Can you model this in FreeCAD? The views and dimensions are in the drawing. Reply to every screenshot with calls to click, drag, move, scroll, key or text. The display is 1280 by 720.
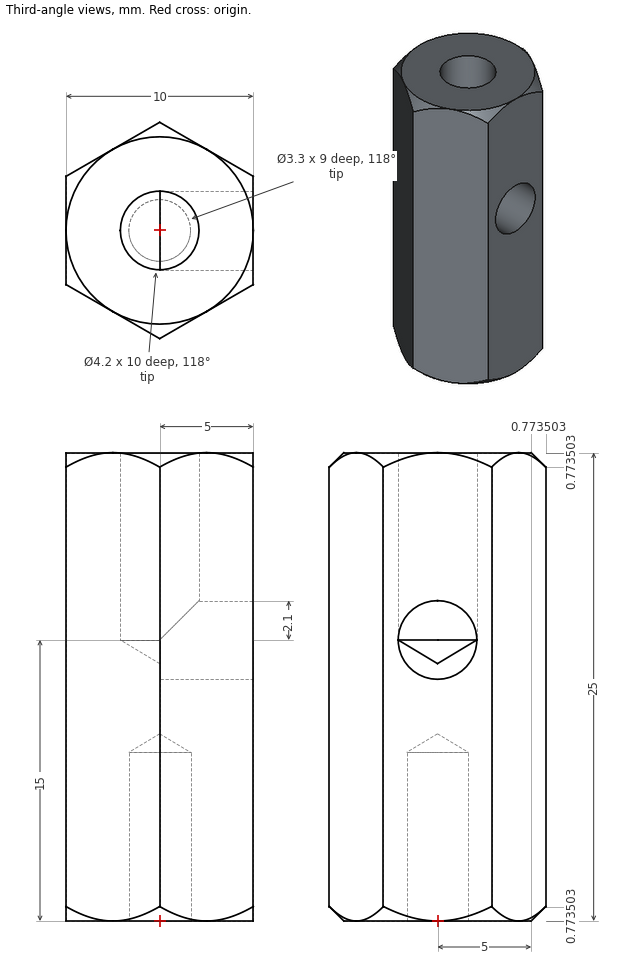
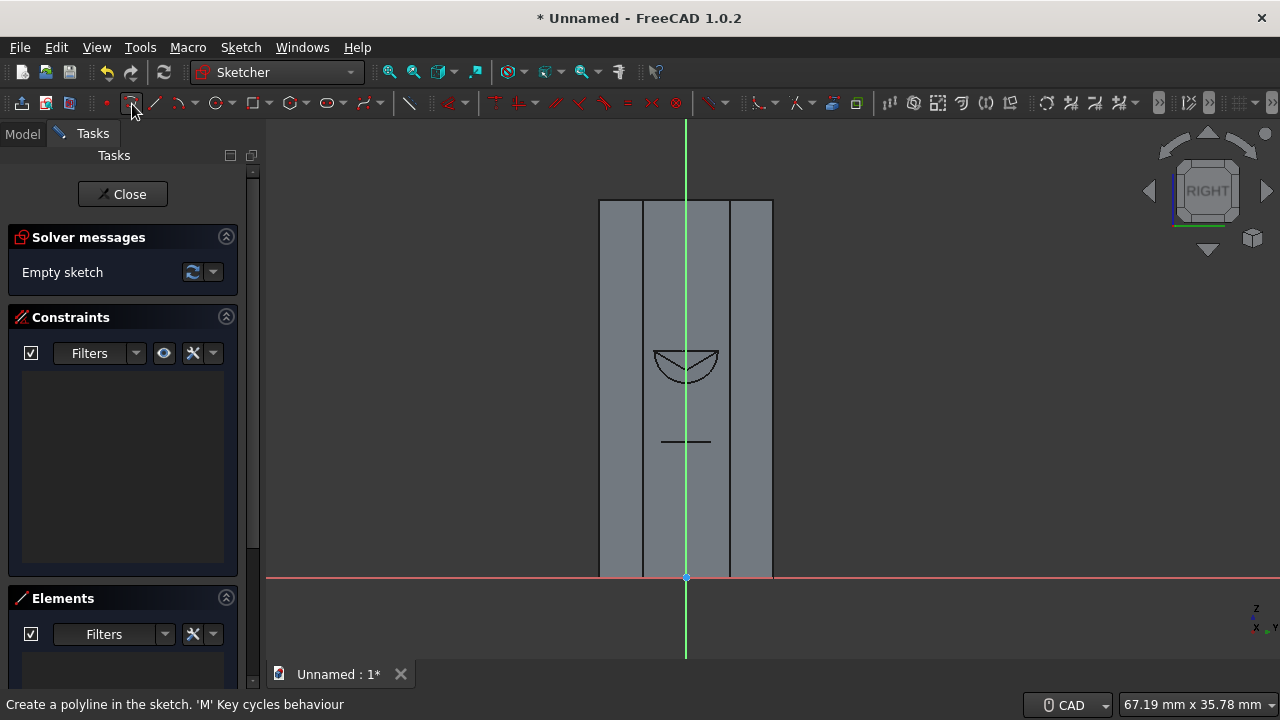
click(773, 212)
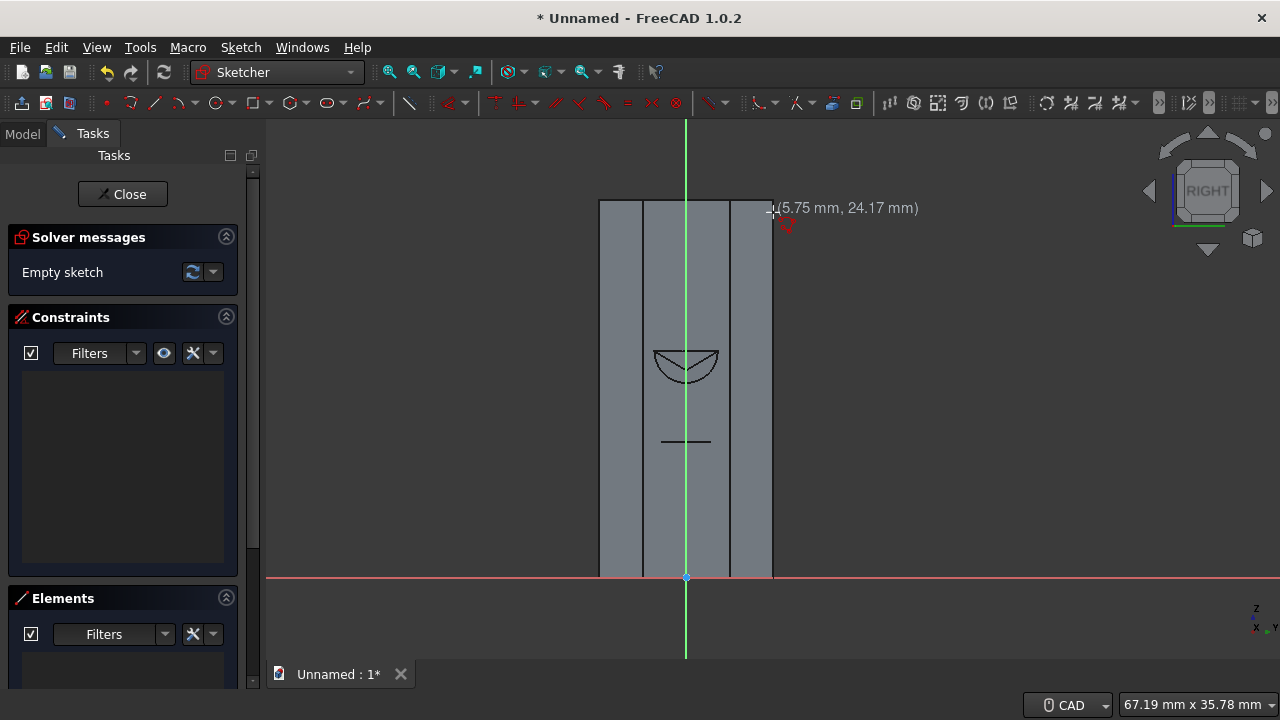
scroll(773, 200, up, 2)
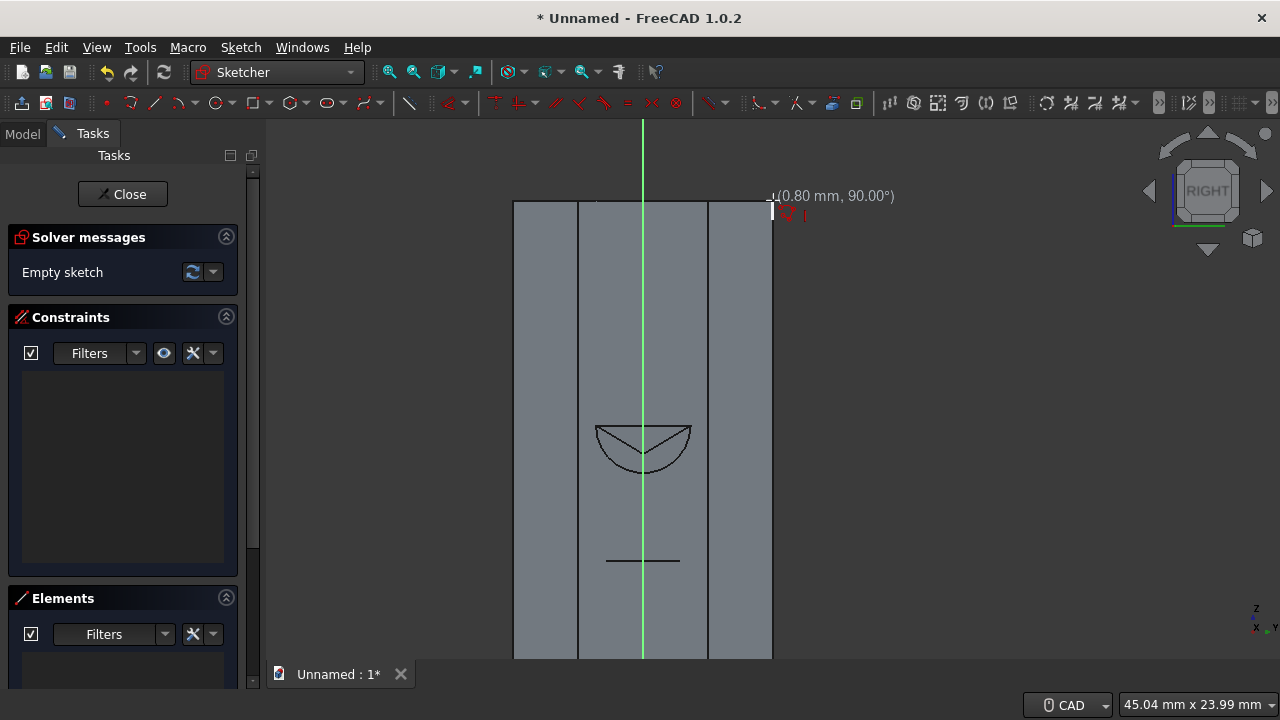
click(773, 201)
click(756, 201)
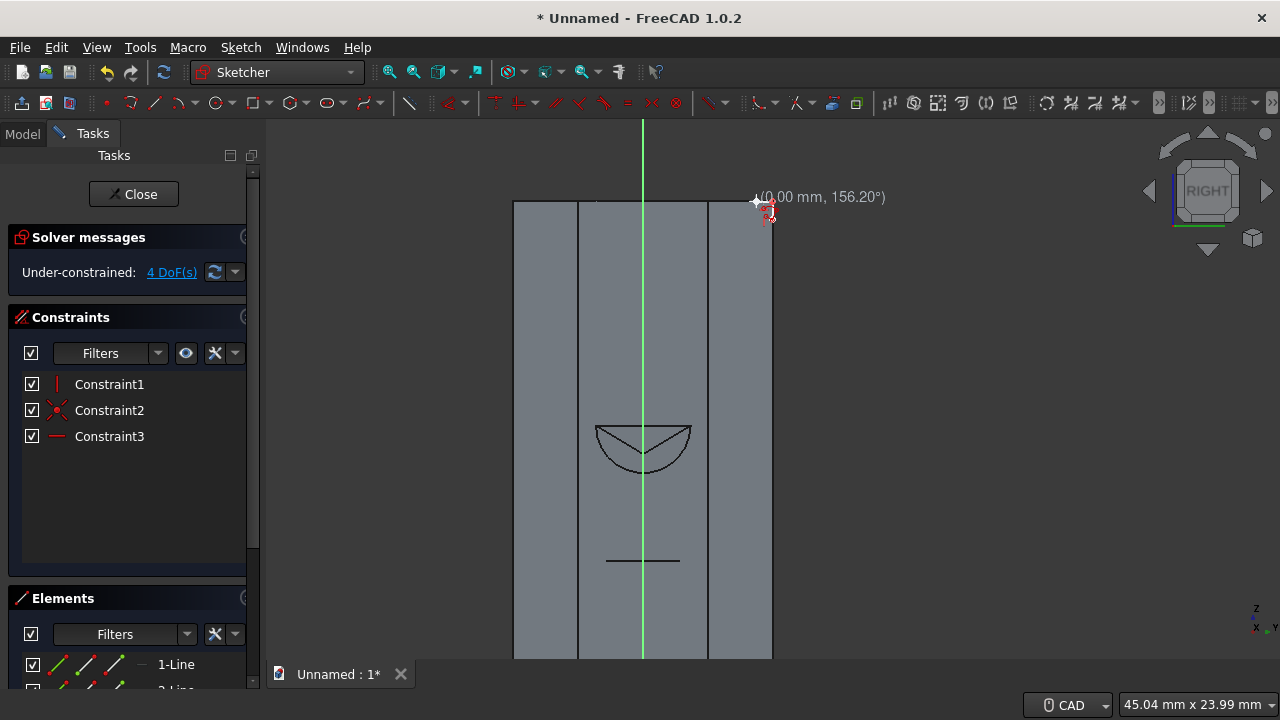
scroll(773, 218, up, 4)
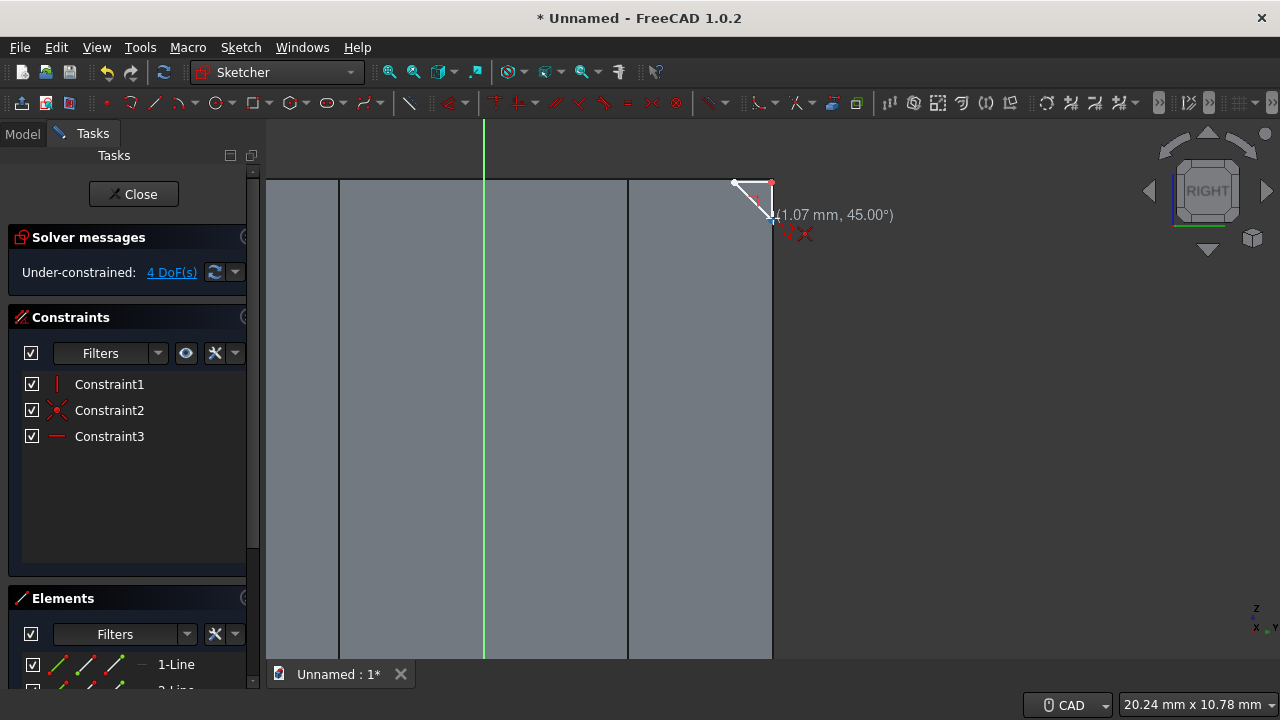
click(772, 221)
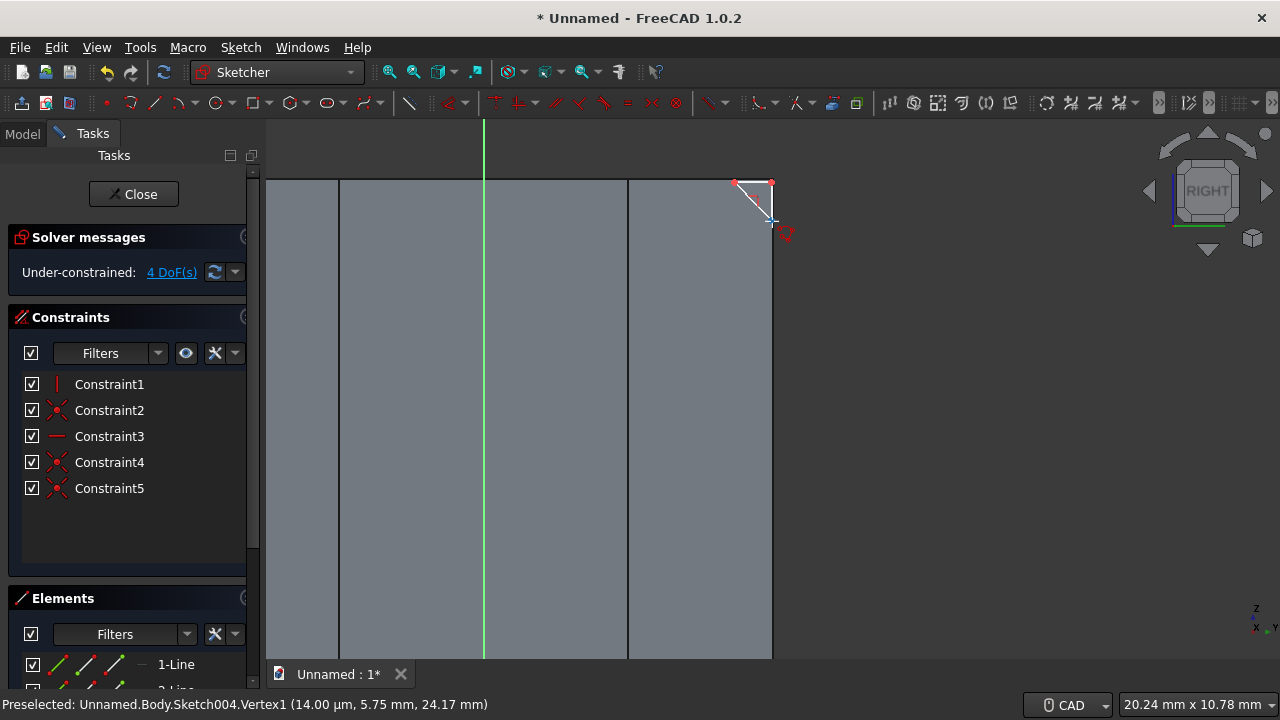
scroll(737, 210, down, 6)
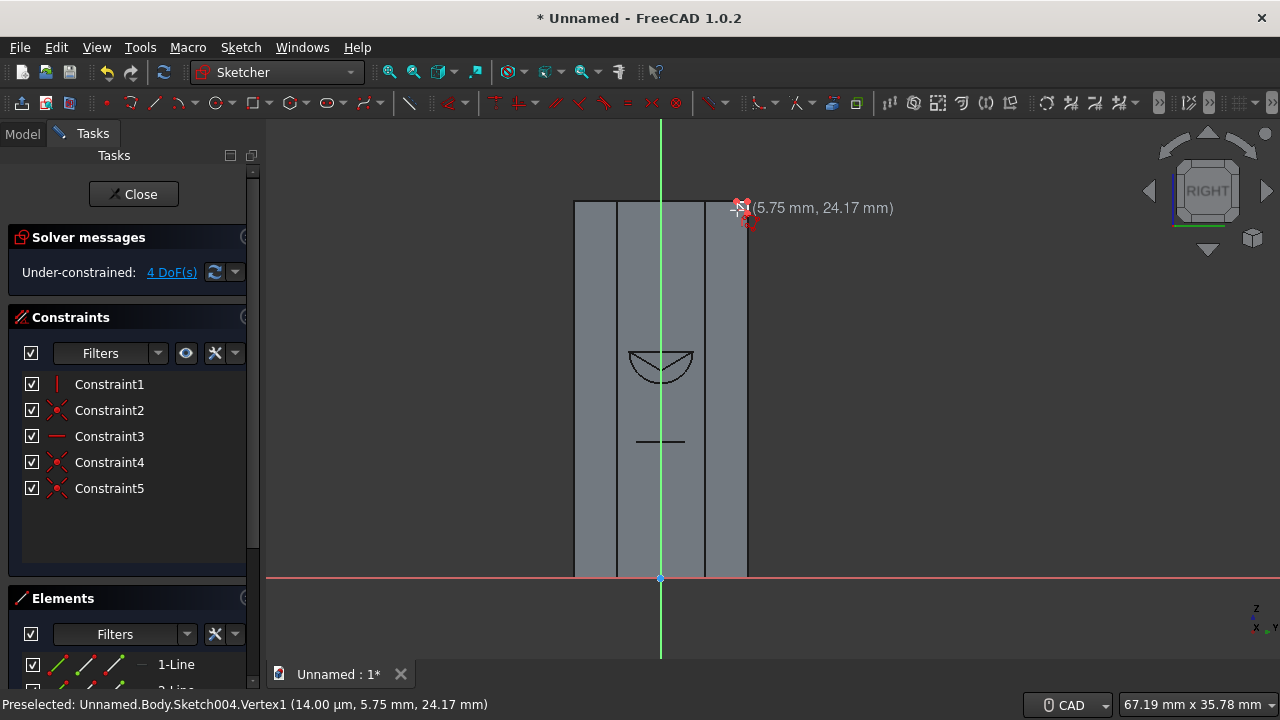
click(736, 578)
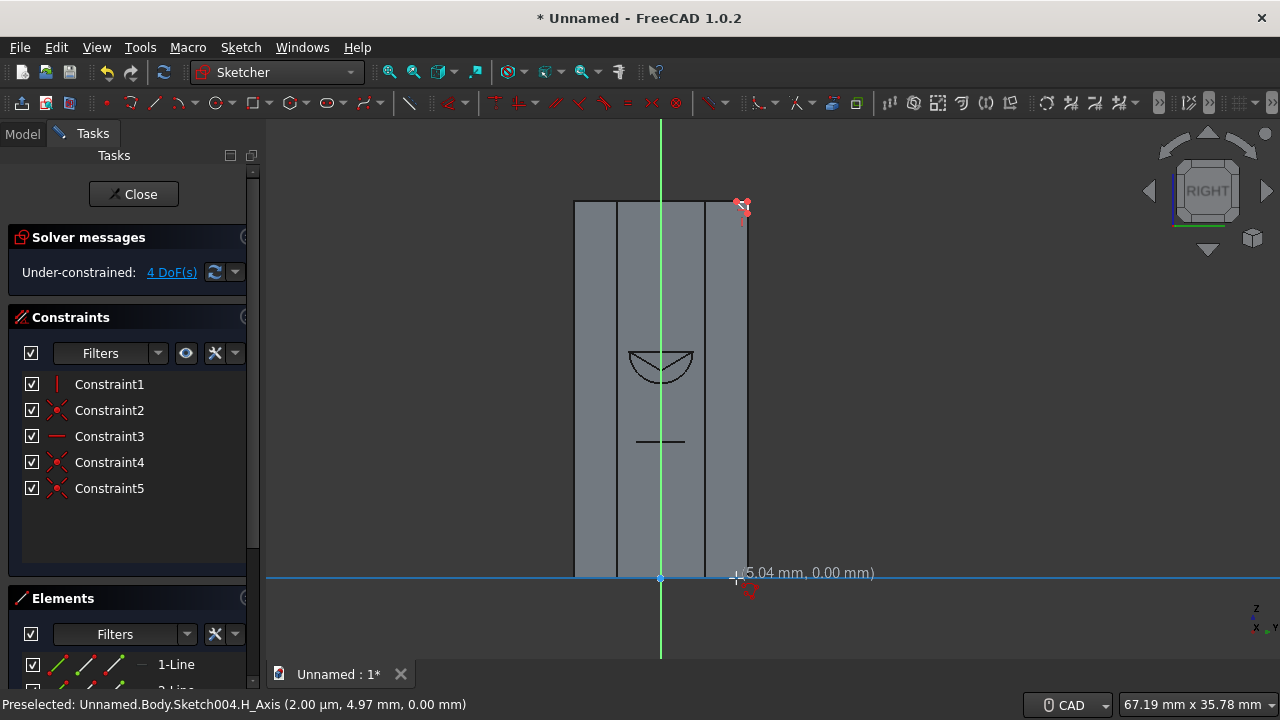
scroll(748, 578, up, 2)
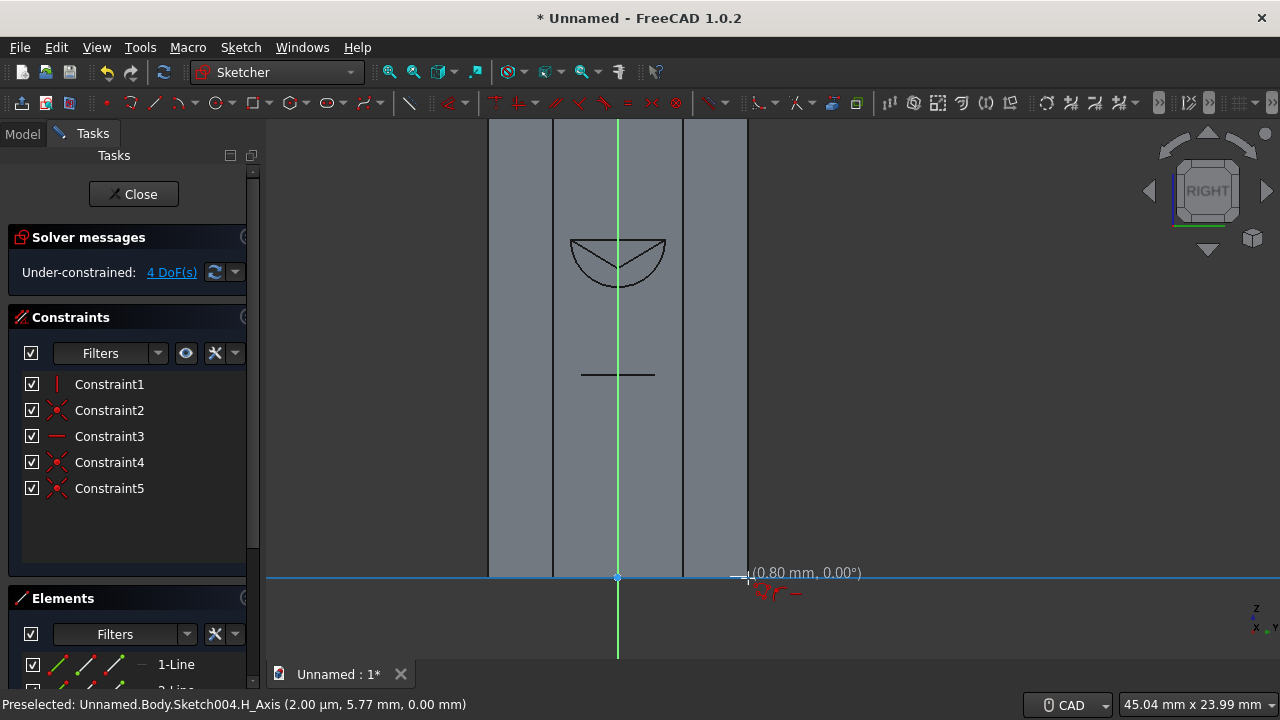
click(748, 569)
click(748, 560)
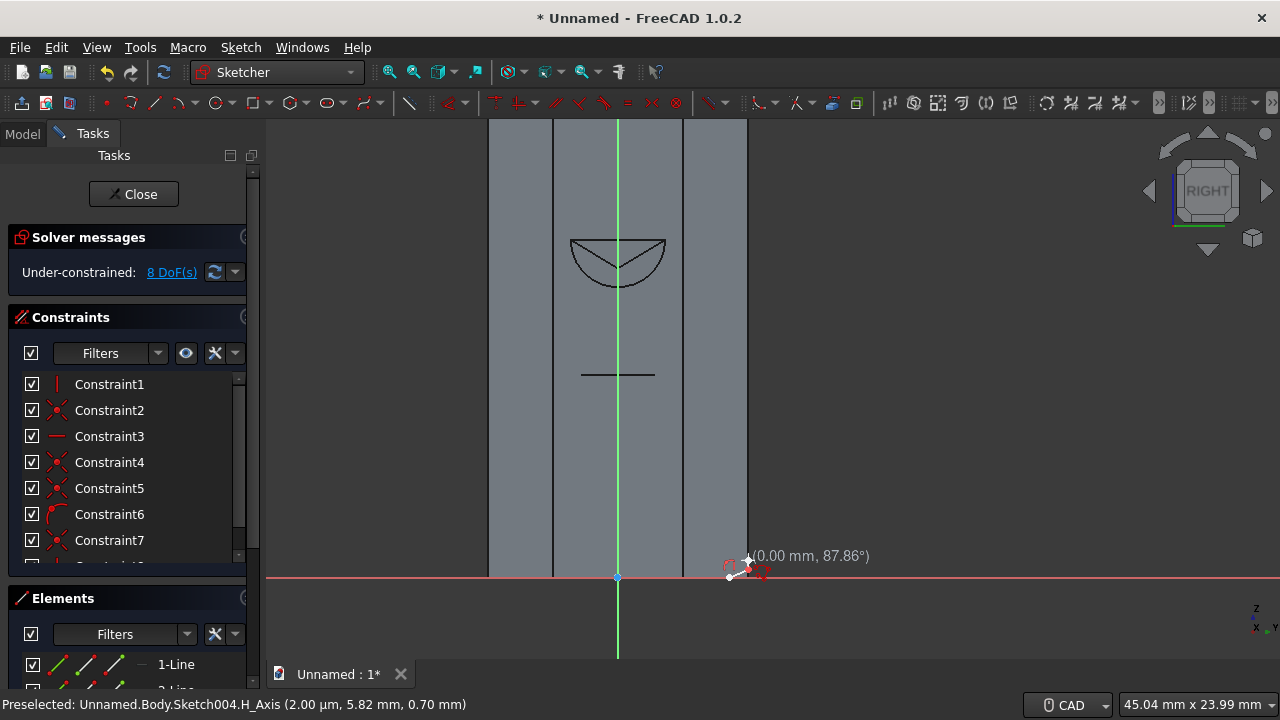
scroll(731, 578, up, 4)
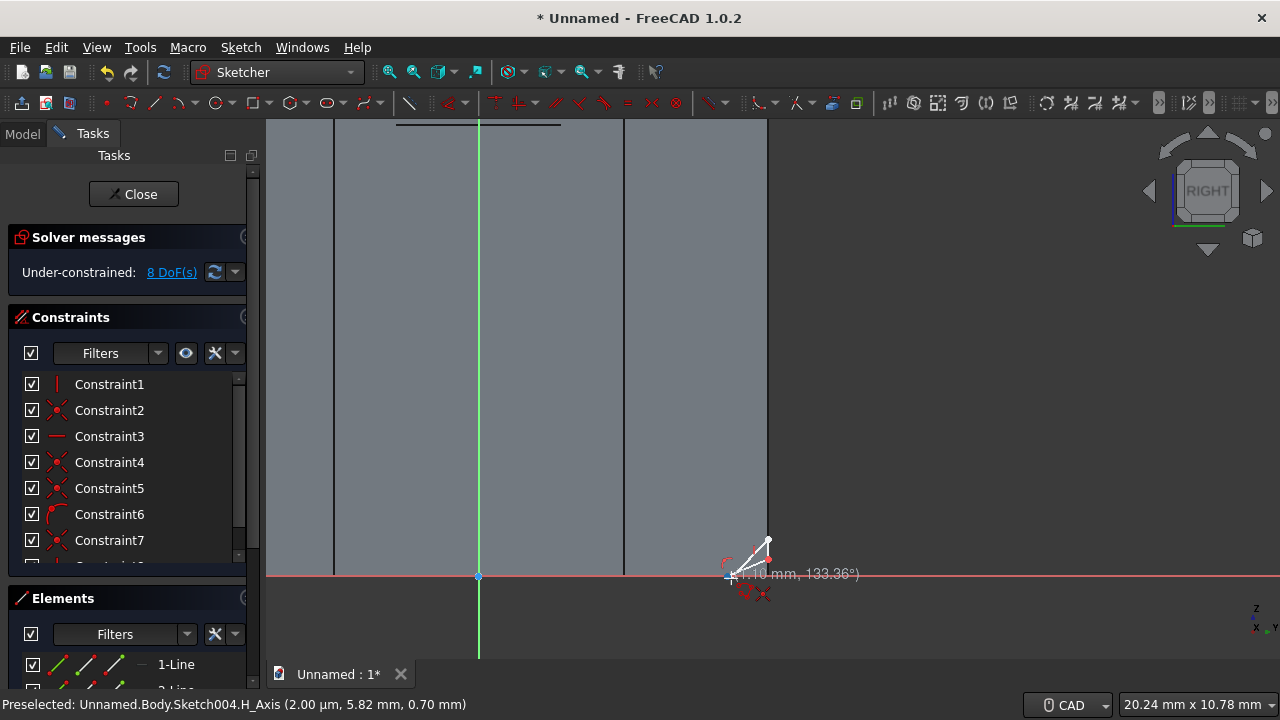
click(728, 576)
key(Escape)
key(Escape)